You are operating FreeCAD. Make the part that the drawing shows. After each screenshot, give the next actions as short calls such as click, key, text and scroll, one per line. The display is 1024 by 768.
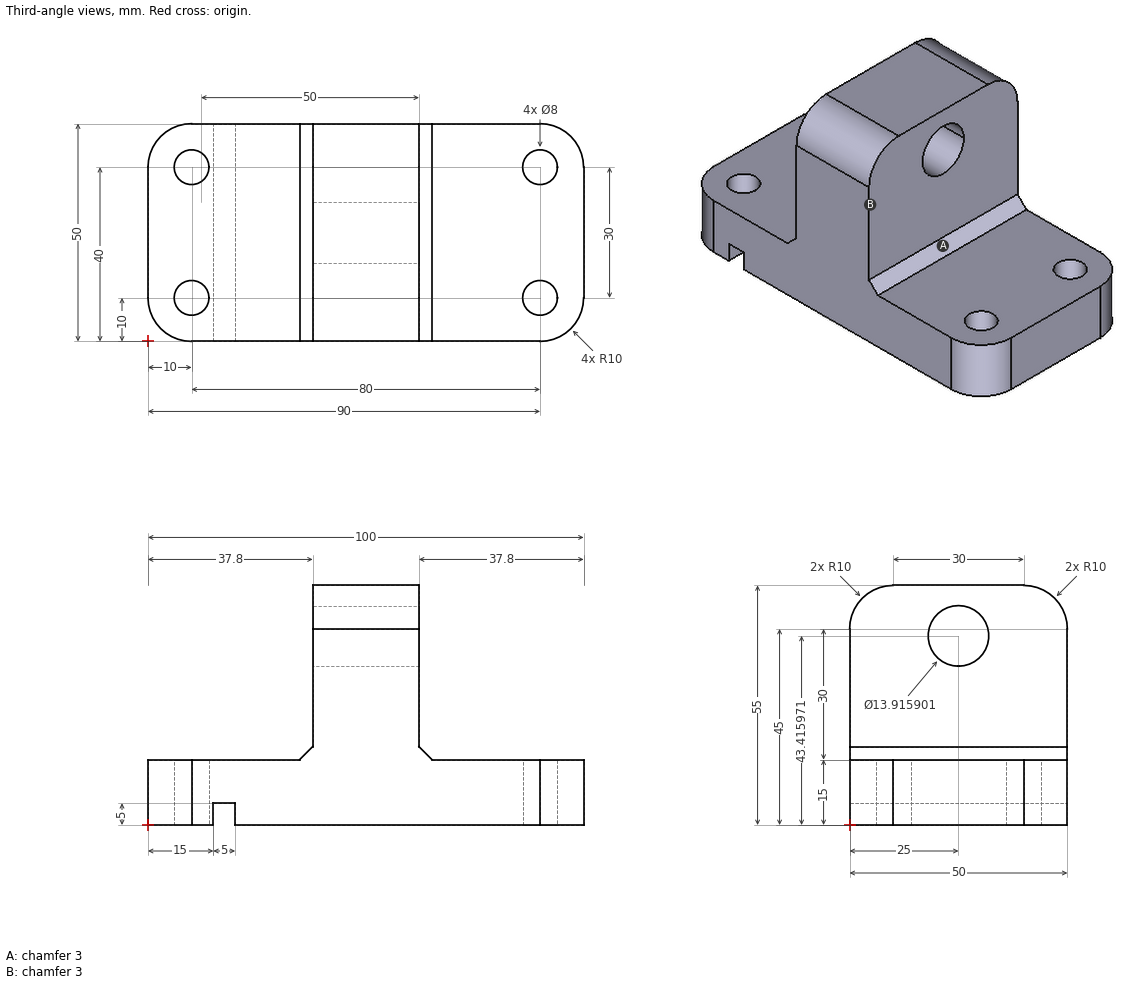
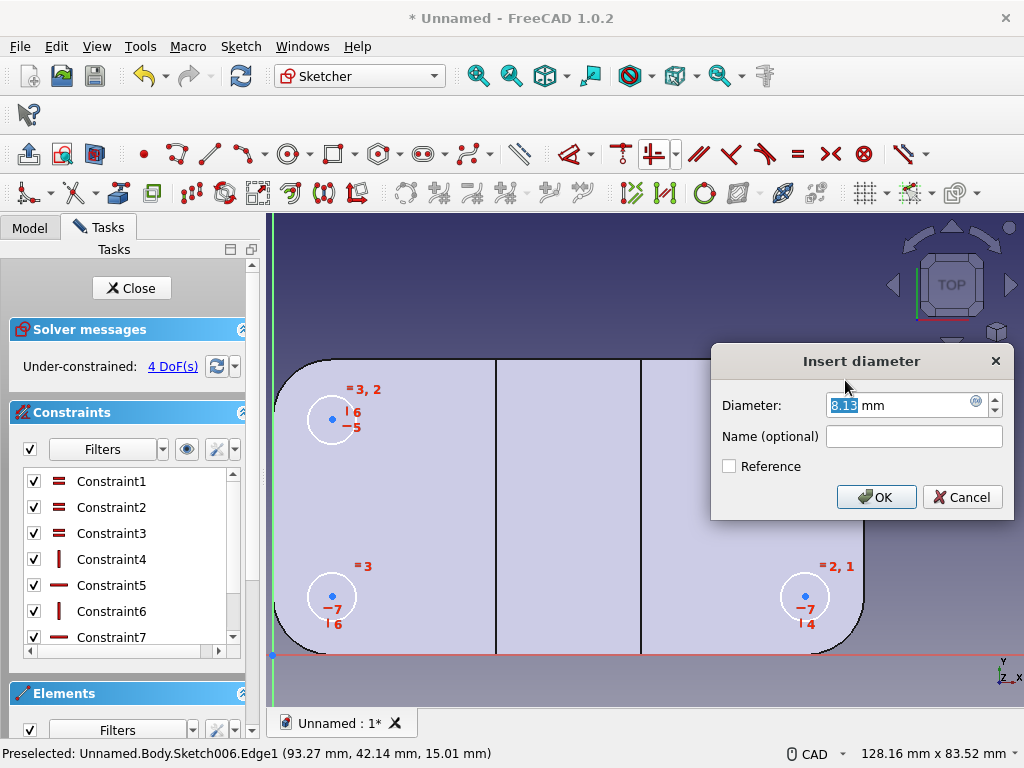
text(8)
key(Return)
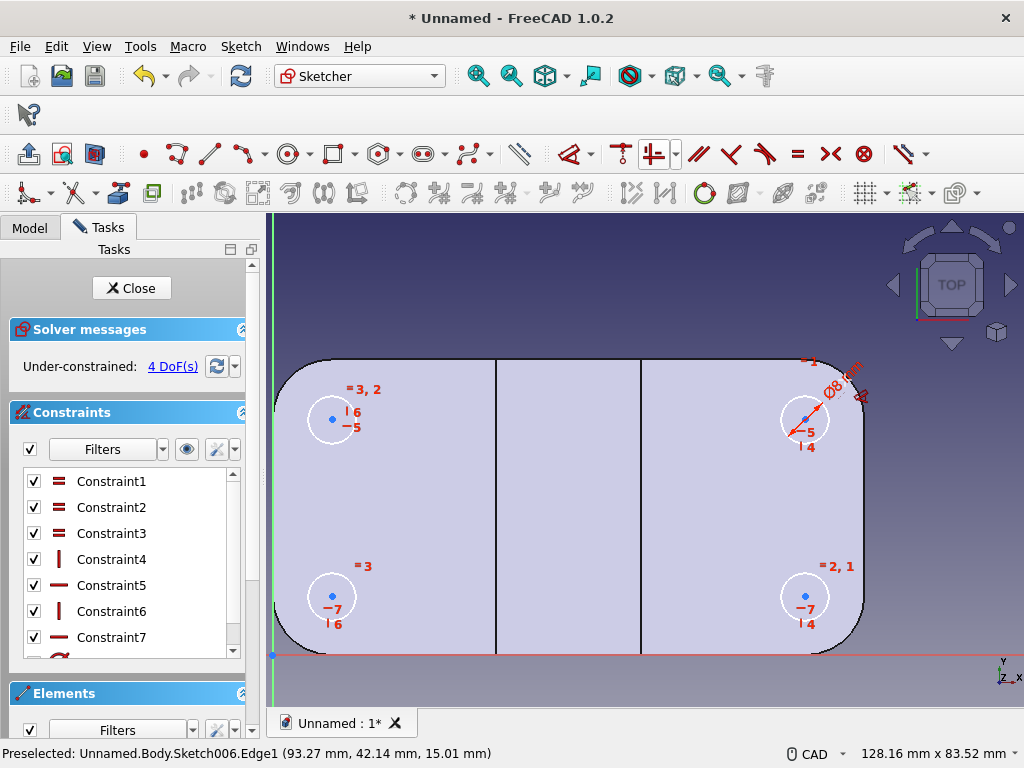
click(805, 420)
click(550, 386)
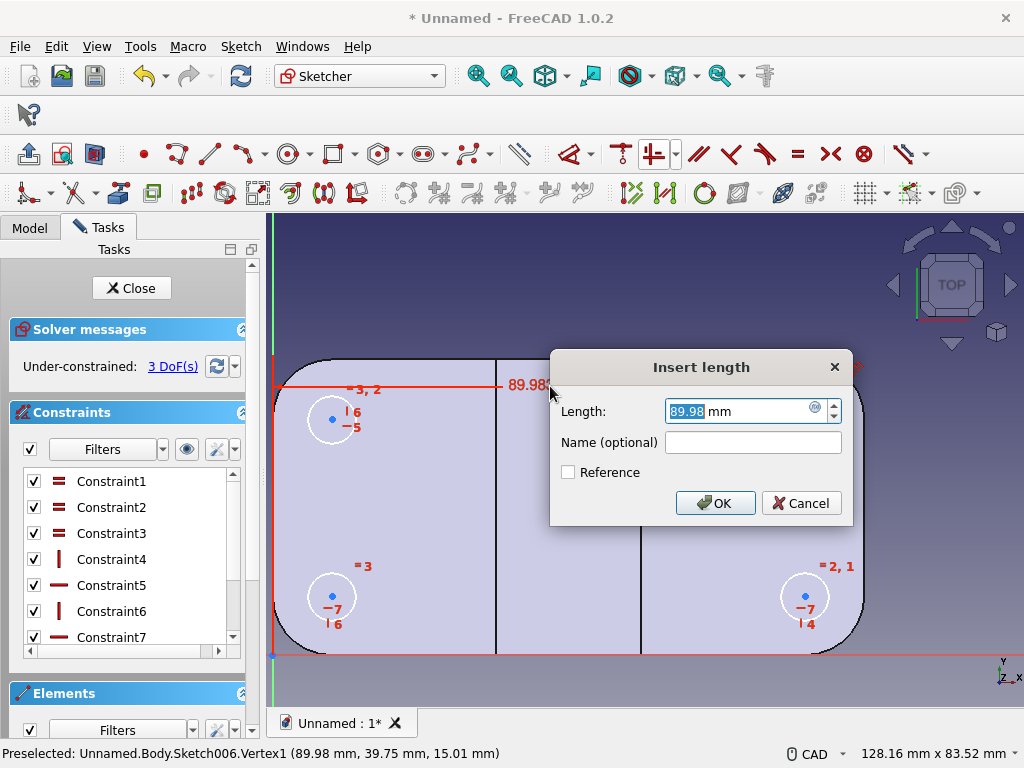
text(90)
key(Return)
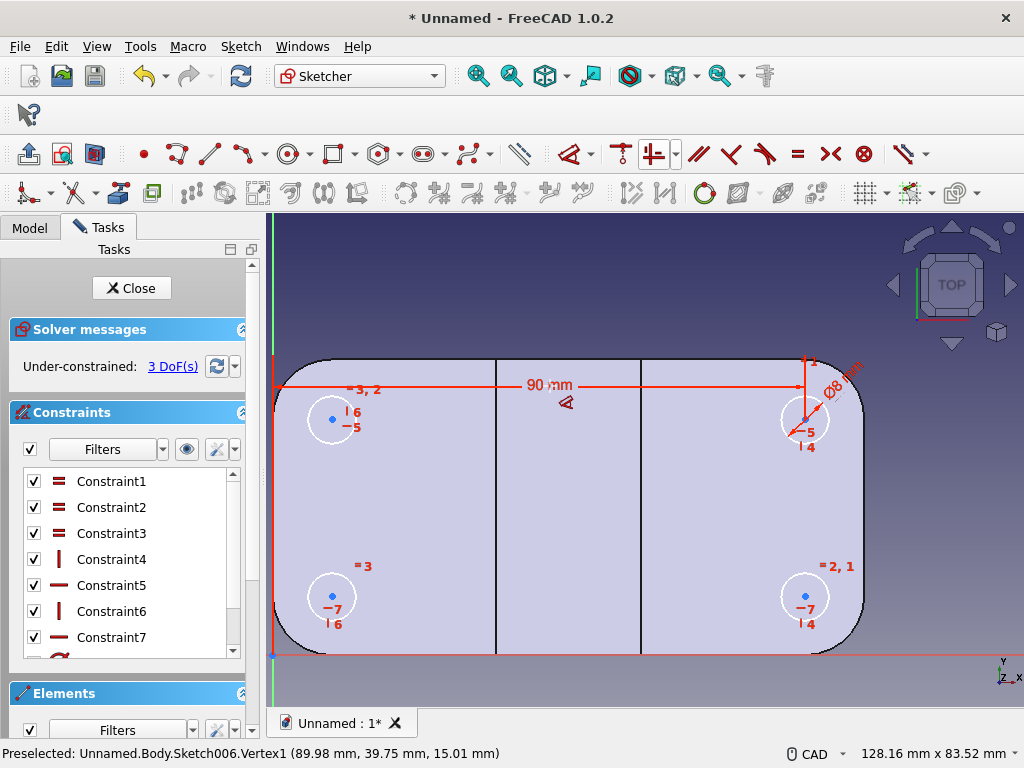
click(805, 420)
click(839, 538)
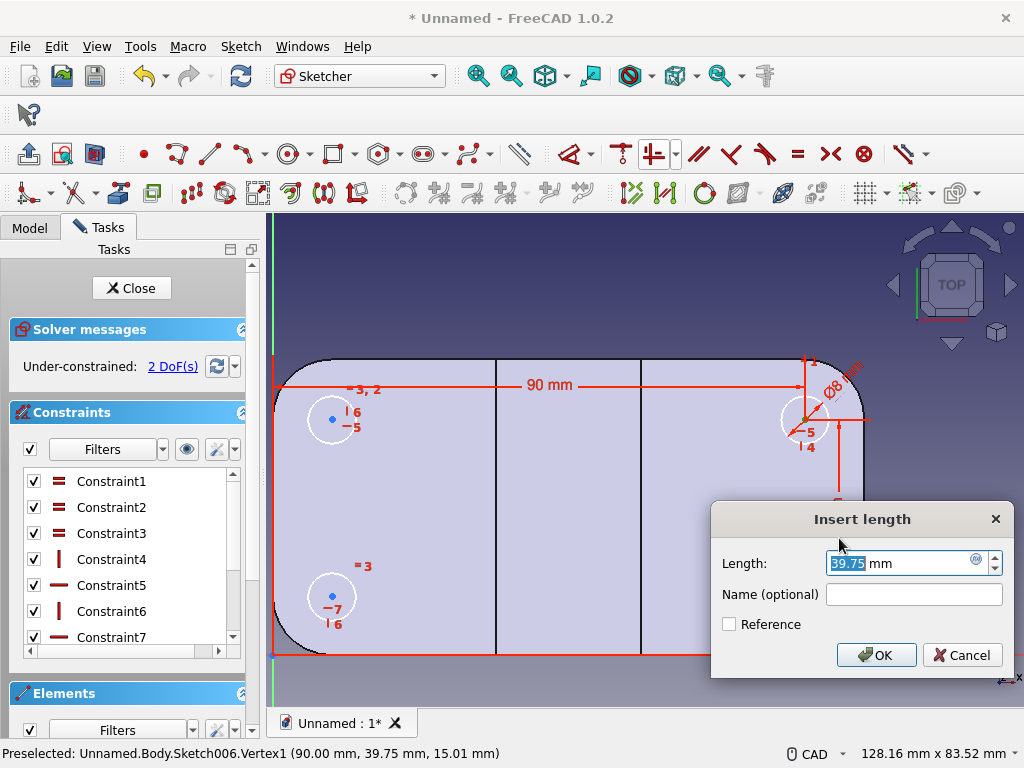
text(40)
key(Return)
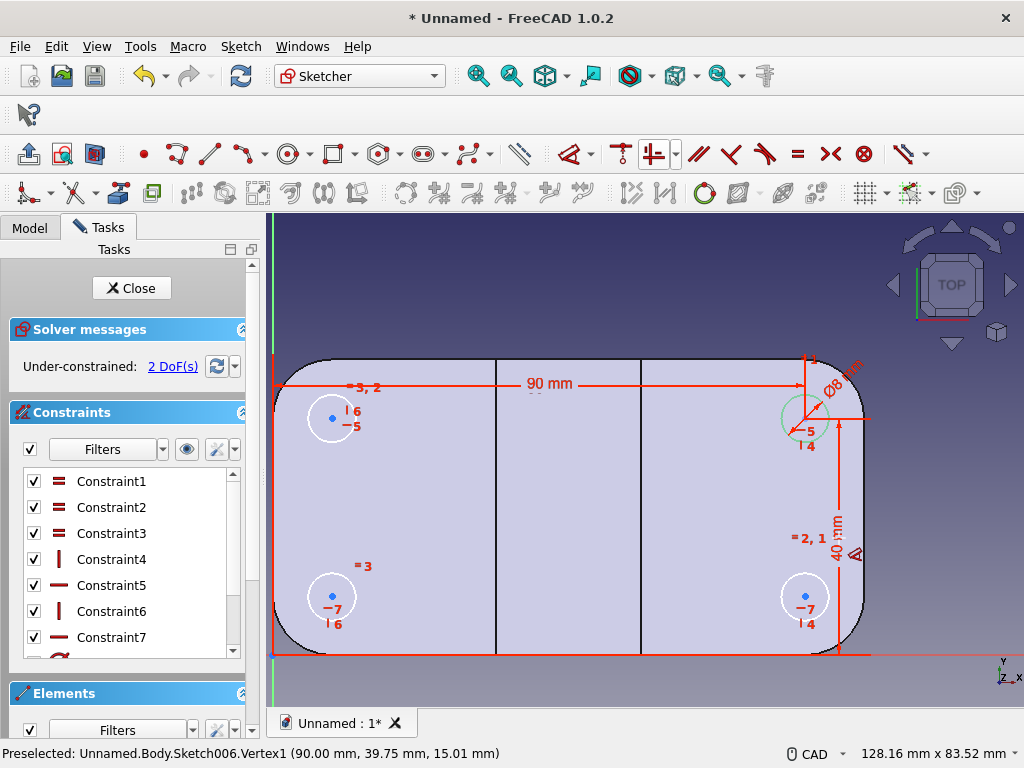
click(805, 597)
click(839, 626)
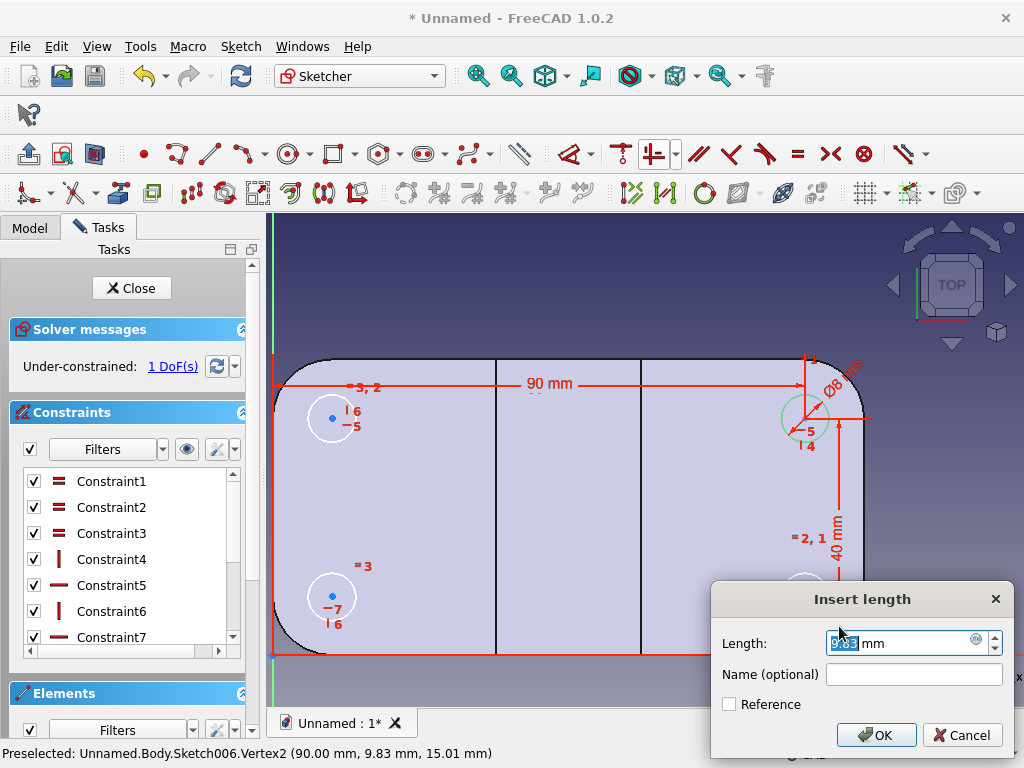
text(10)
key(Return)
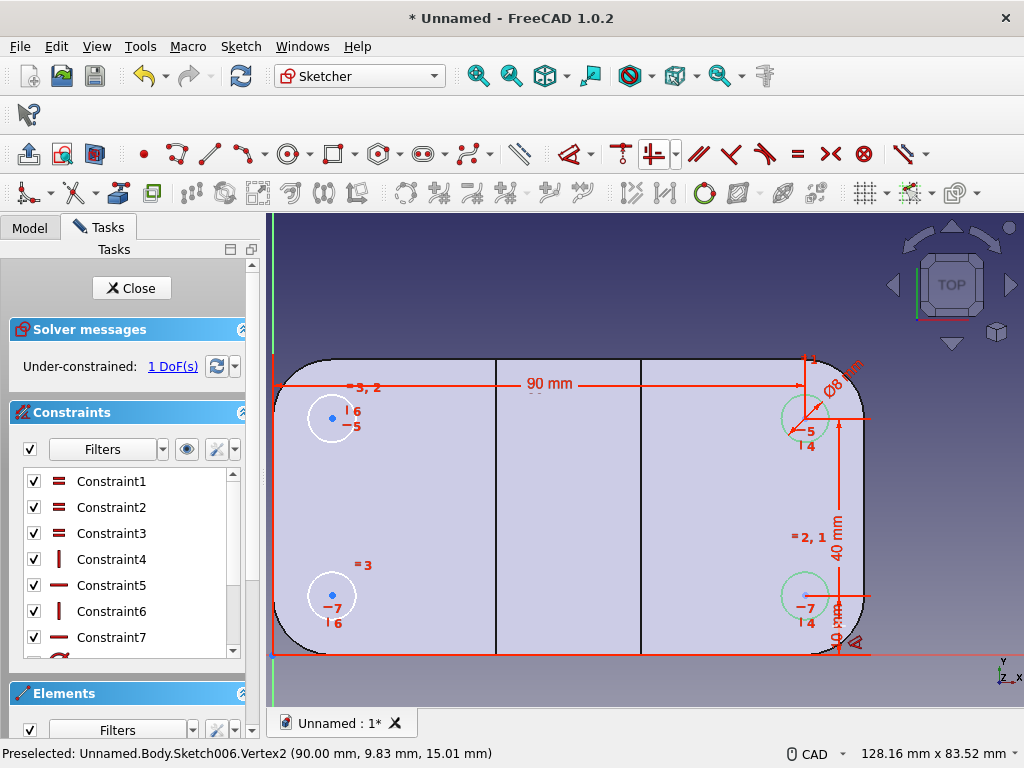
click(332, 419)
click(313, 385)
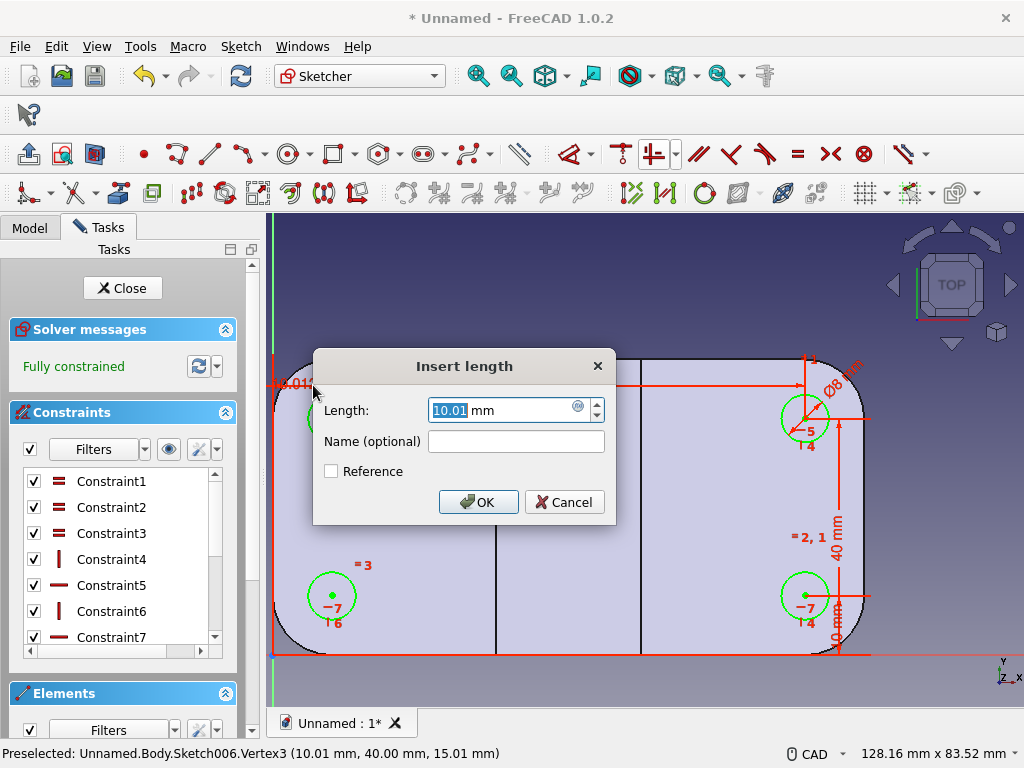
text(10)
key(Return)
key(Escape)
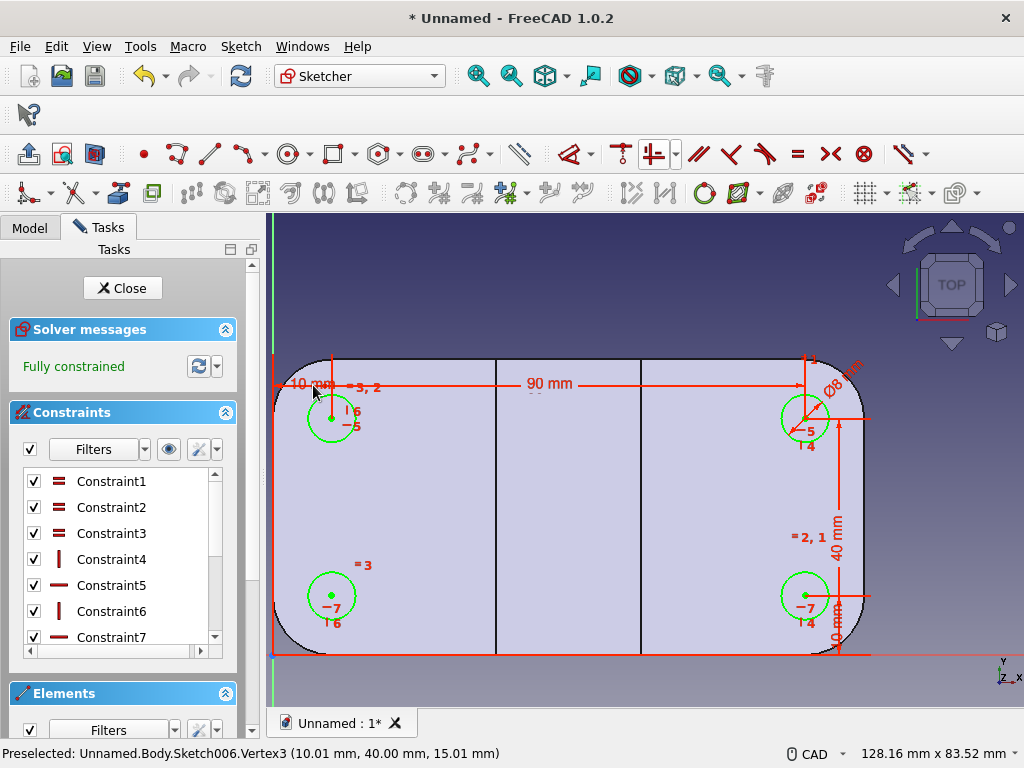
click(123, 288)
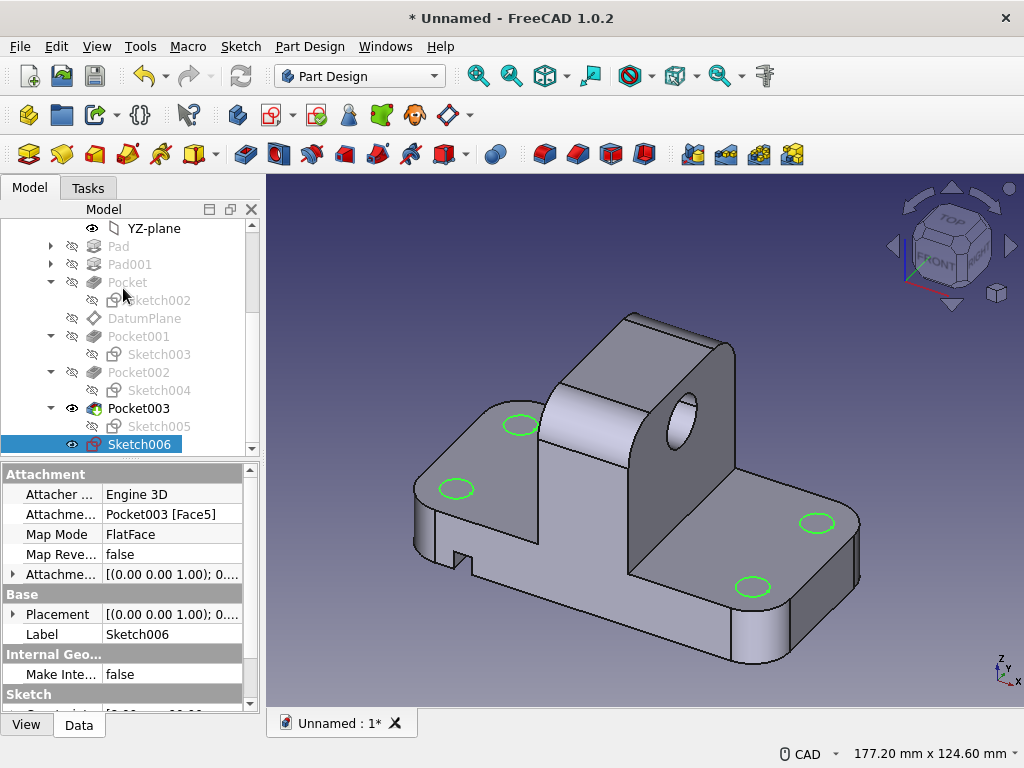
click(246, 154)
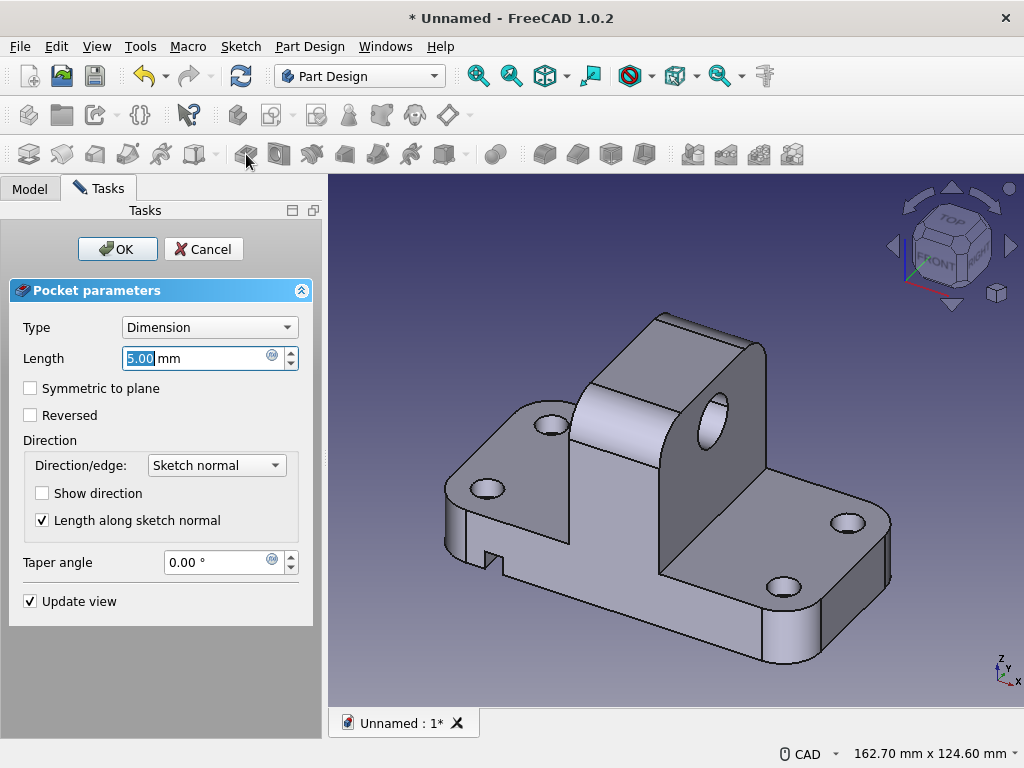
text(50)
key(Tab)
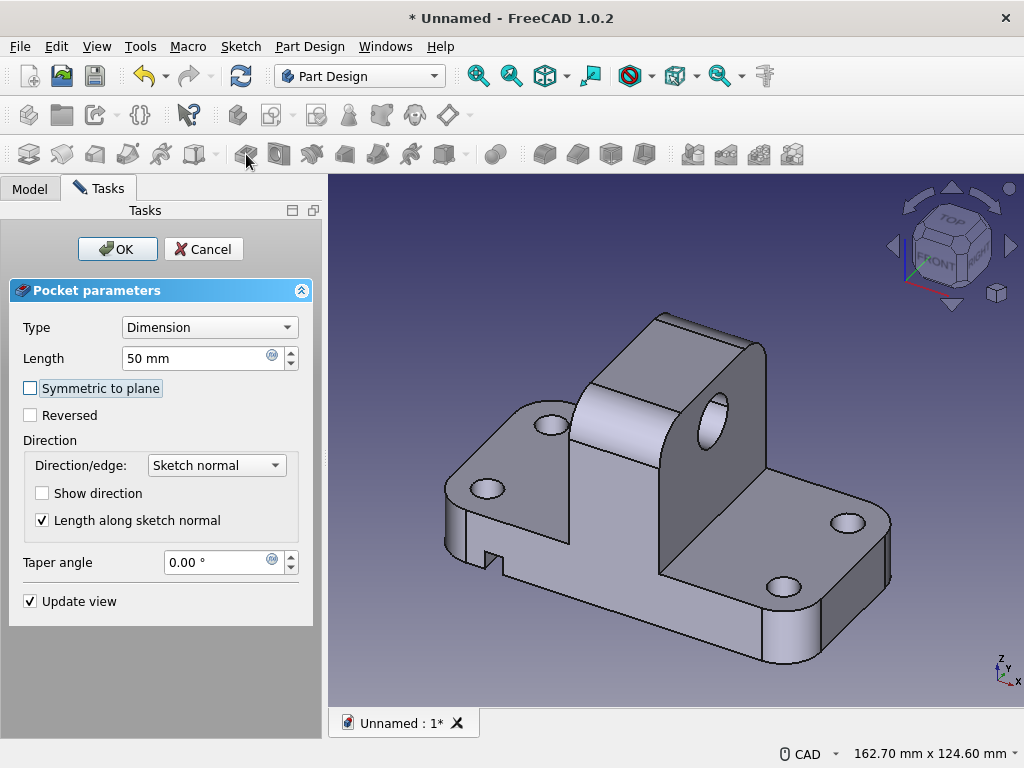
click(118, 249)